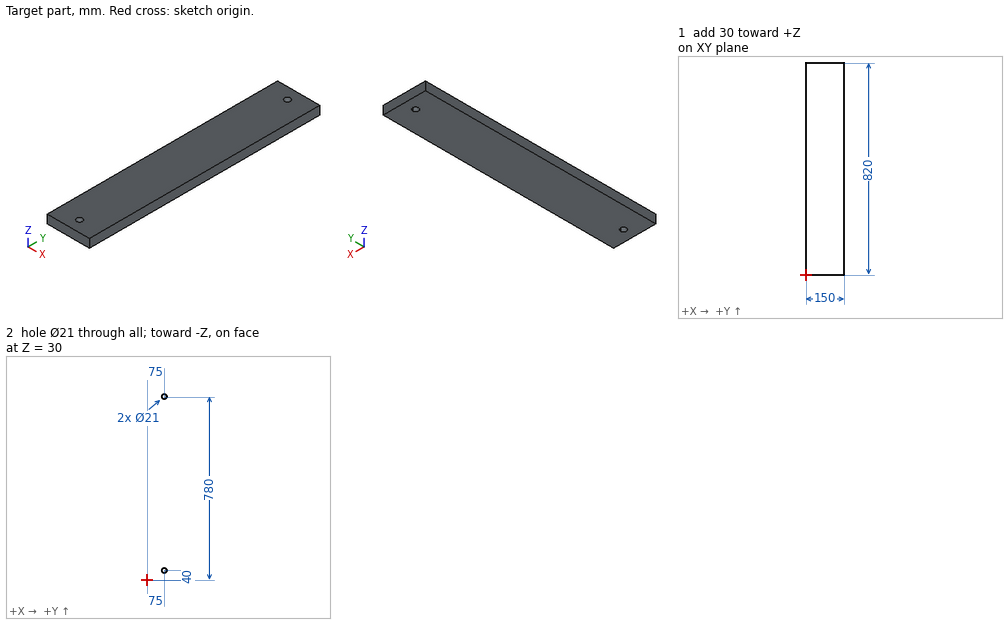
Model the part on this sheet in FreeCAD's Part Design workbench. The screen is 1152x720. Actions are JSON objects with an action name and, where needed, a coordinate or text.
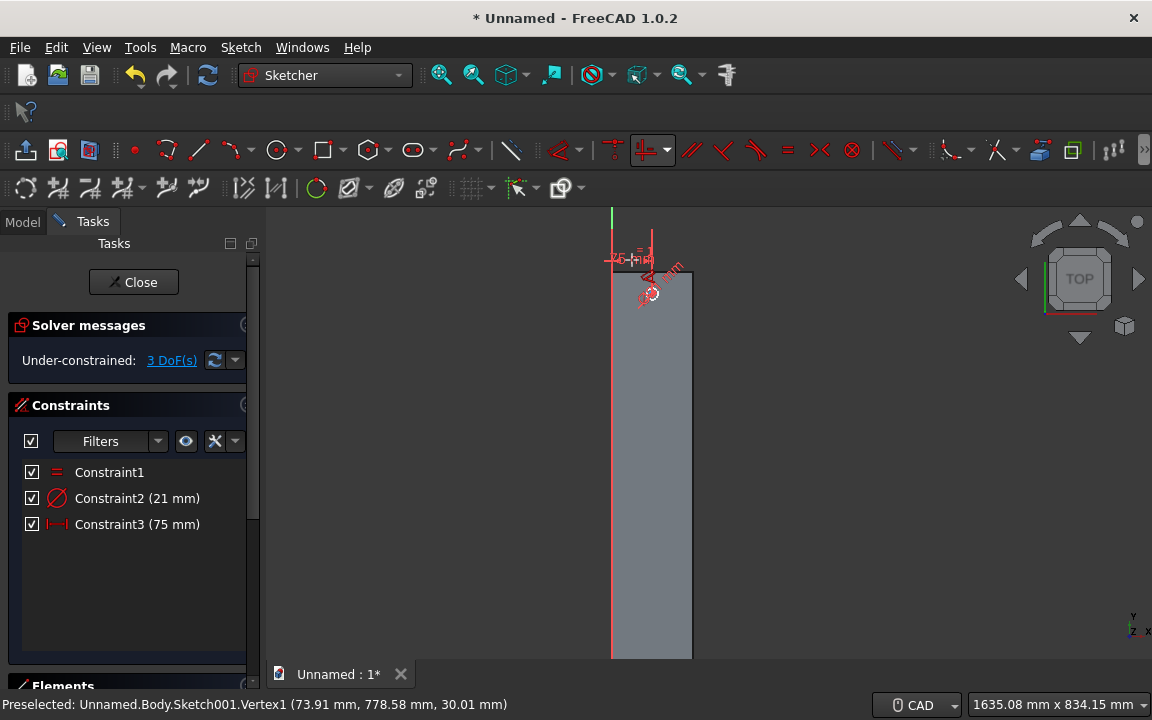
{"action": "scroll", "coordinate": [652, 293], "scroll_direction": "down", "scroll_amount": 2}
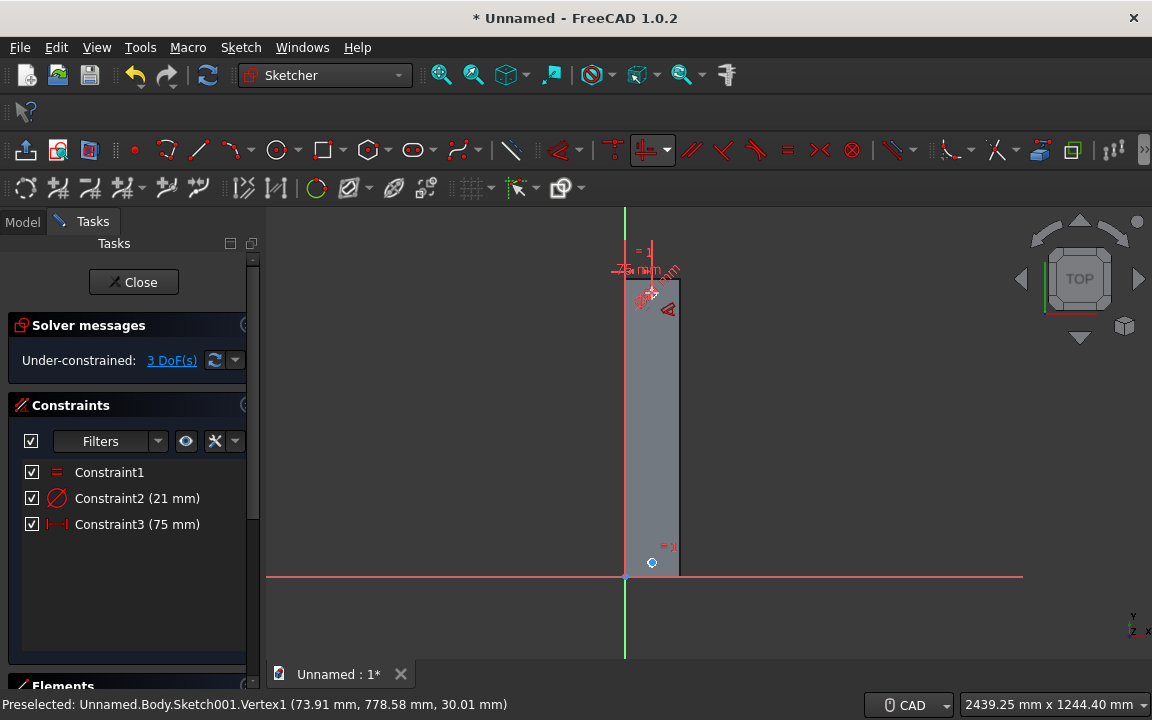
{"action": "scroll", "coordinate": [652, 563], "scroll_direction": "up", "scroll_amount": 2}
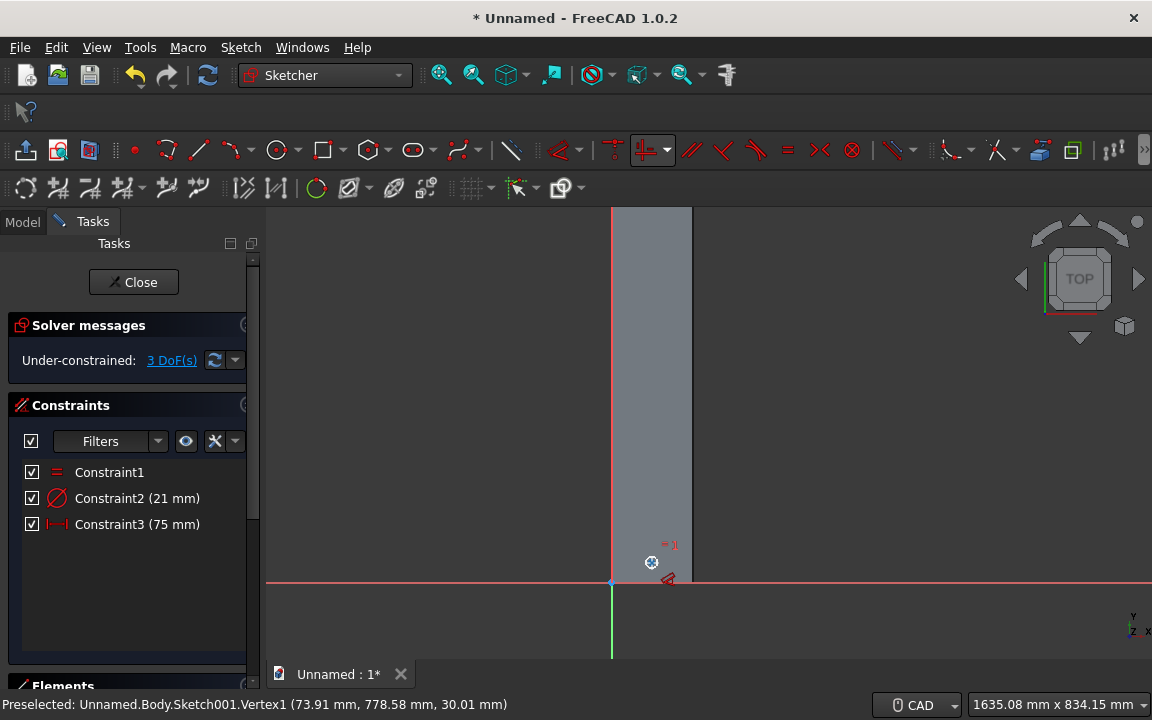
{"action": "left_click", "coordinate": [652, 562]}
{"action": "left_click", "coordinate": [632, 617]}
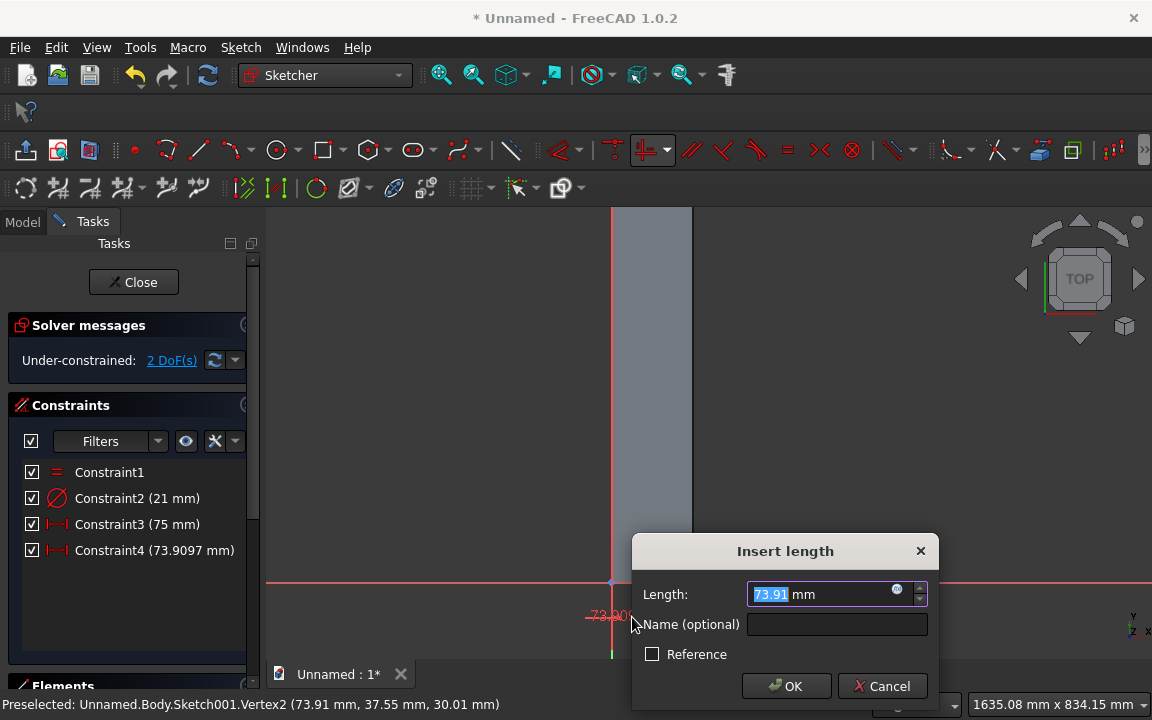
{"action": "type", "text": "75"}
{"action": "key", "text": "Return"}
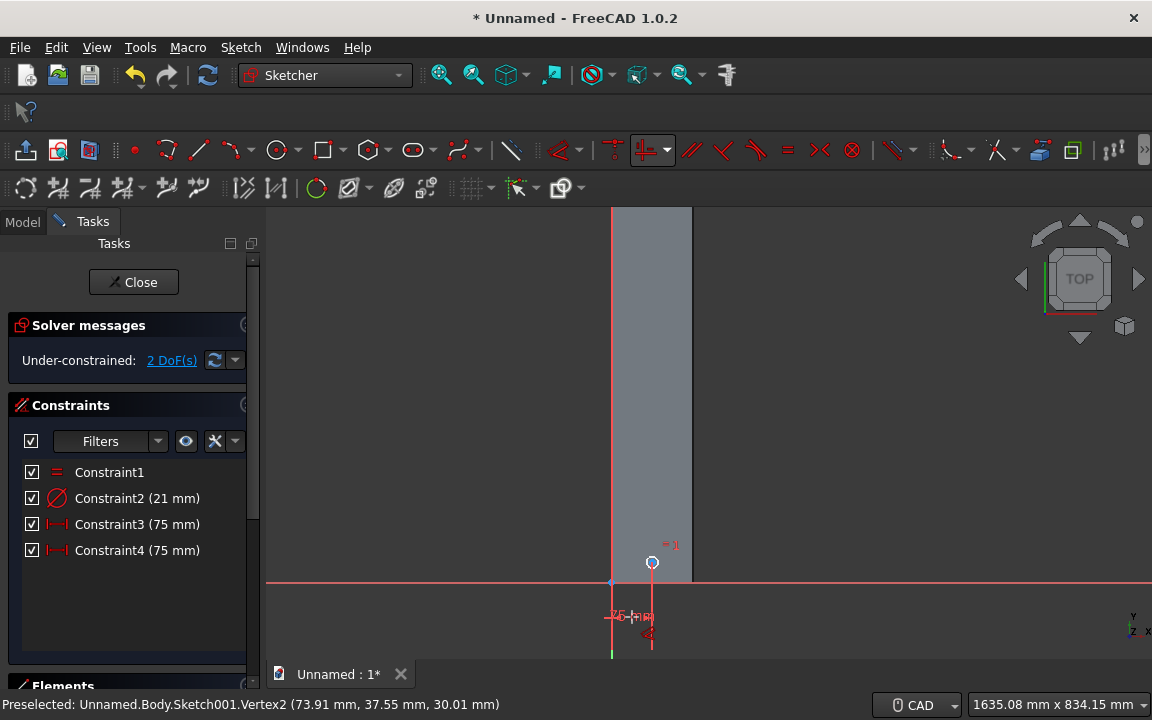
{"action": "scroll", "coordinate": [652, 562], "scroll_direction": "up", "scroll_amount": 4}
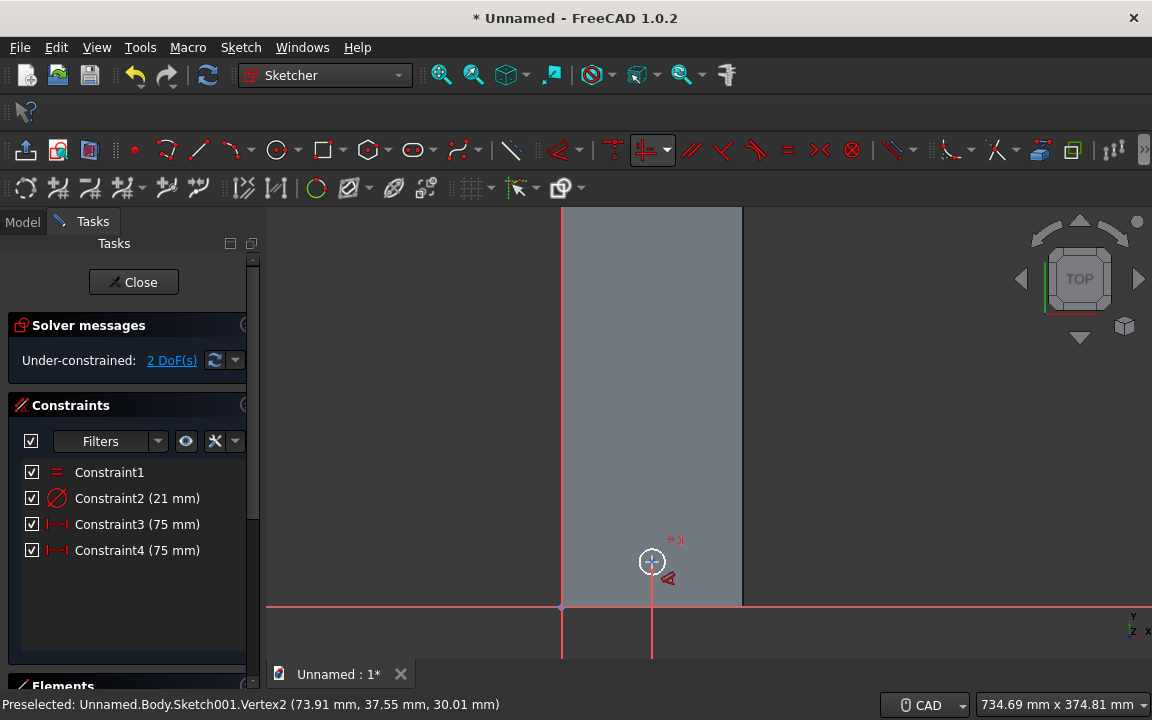
{"action": "left_click", "coordinate": [652, 562]}
{"action": "left_click", "coordinate": [528, 585]}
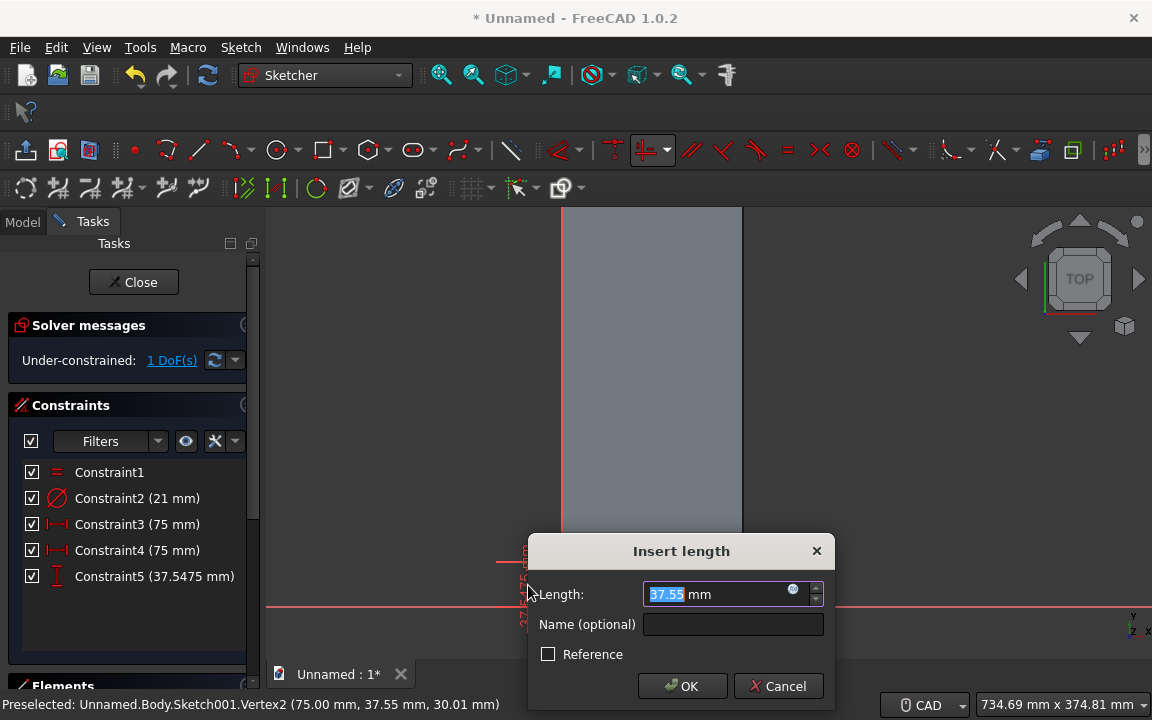
{"action": "type", "text": "40"}
{"action": "key", "text": "Return"}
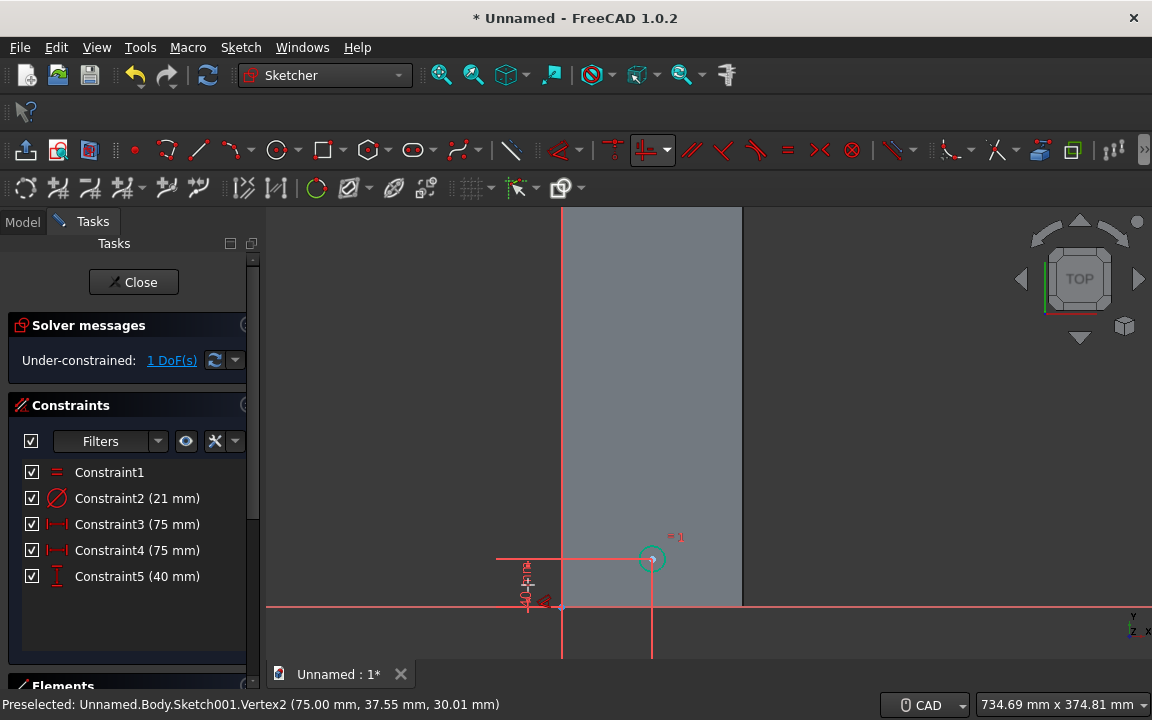
{"action": "scroll", "coordinate": [652, 563], "scroll_direction": "down", "scroll_amount": 6}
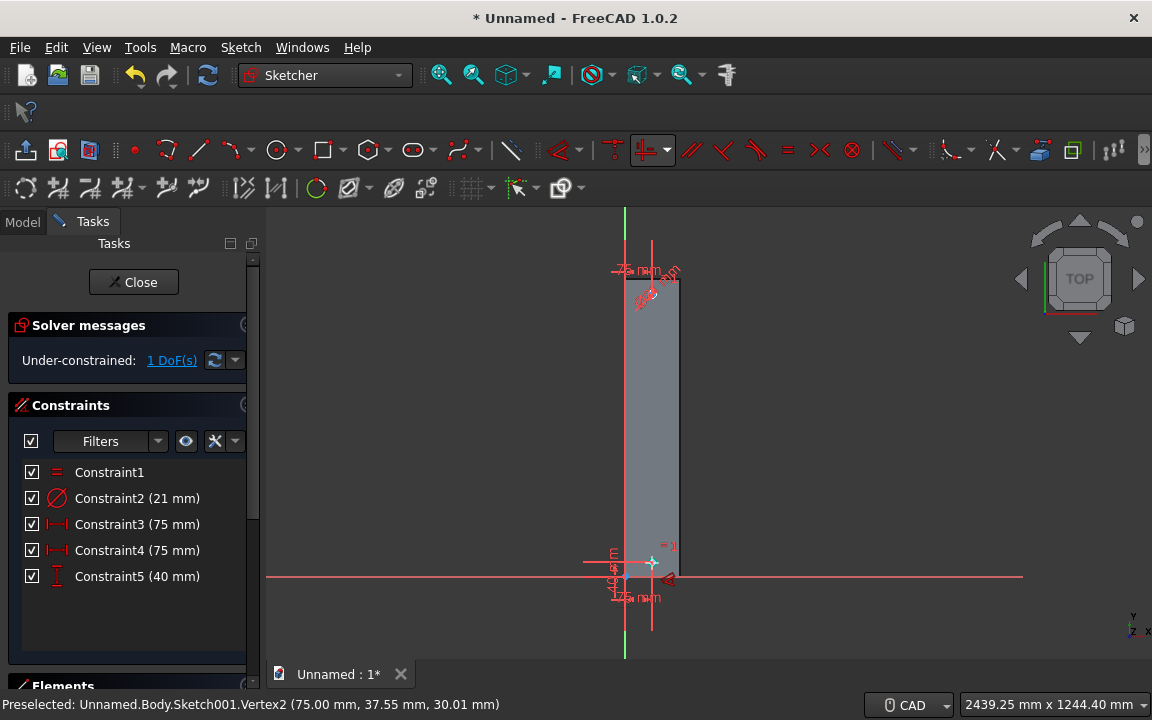
{"action": "left_click", "coordinate": [652, 294]}
{"action": "left_click", "coordinate": [591, 435]}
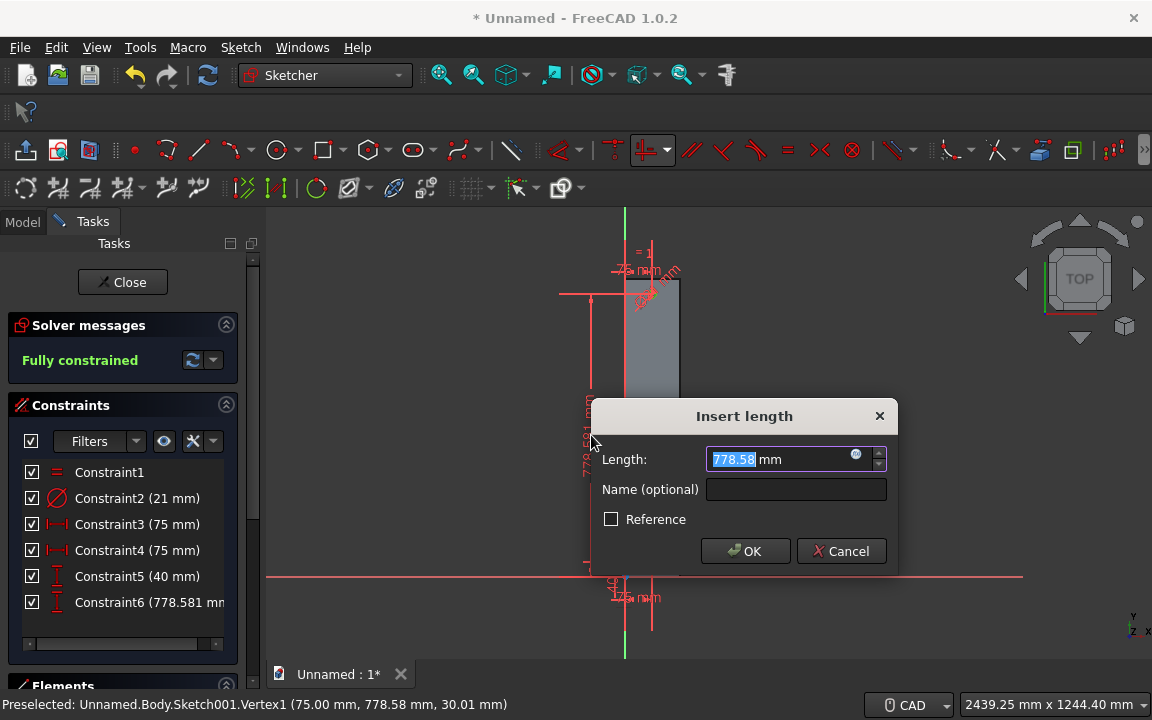
{"action": "type", "text": "780"}
{"action": "key", "text": "Return"}
{"action": "key", "text": "Escape"}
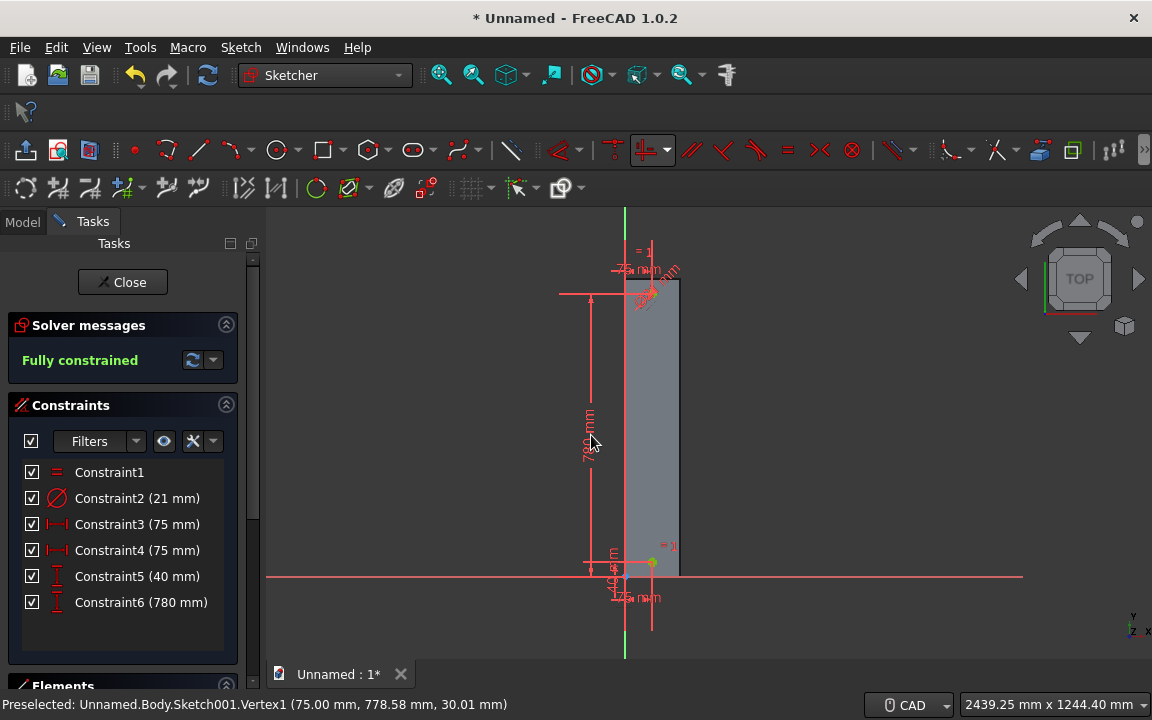
{"action": "left_click", "coordinate": [123, 282]}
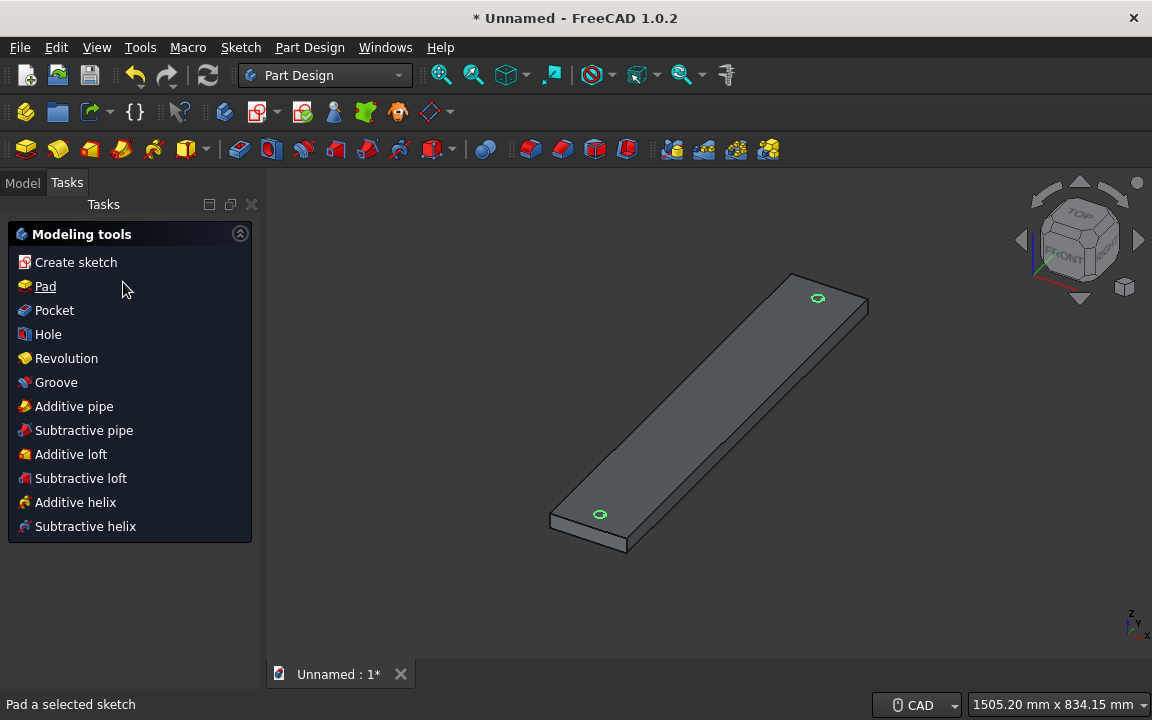
{"action": "left_click", "coordinate": [272, 150]}